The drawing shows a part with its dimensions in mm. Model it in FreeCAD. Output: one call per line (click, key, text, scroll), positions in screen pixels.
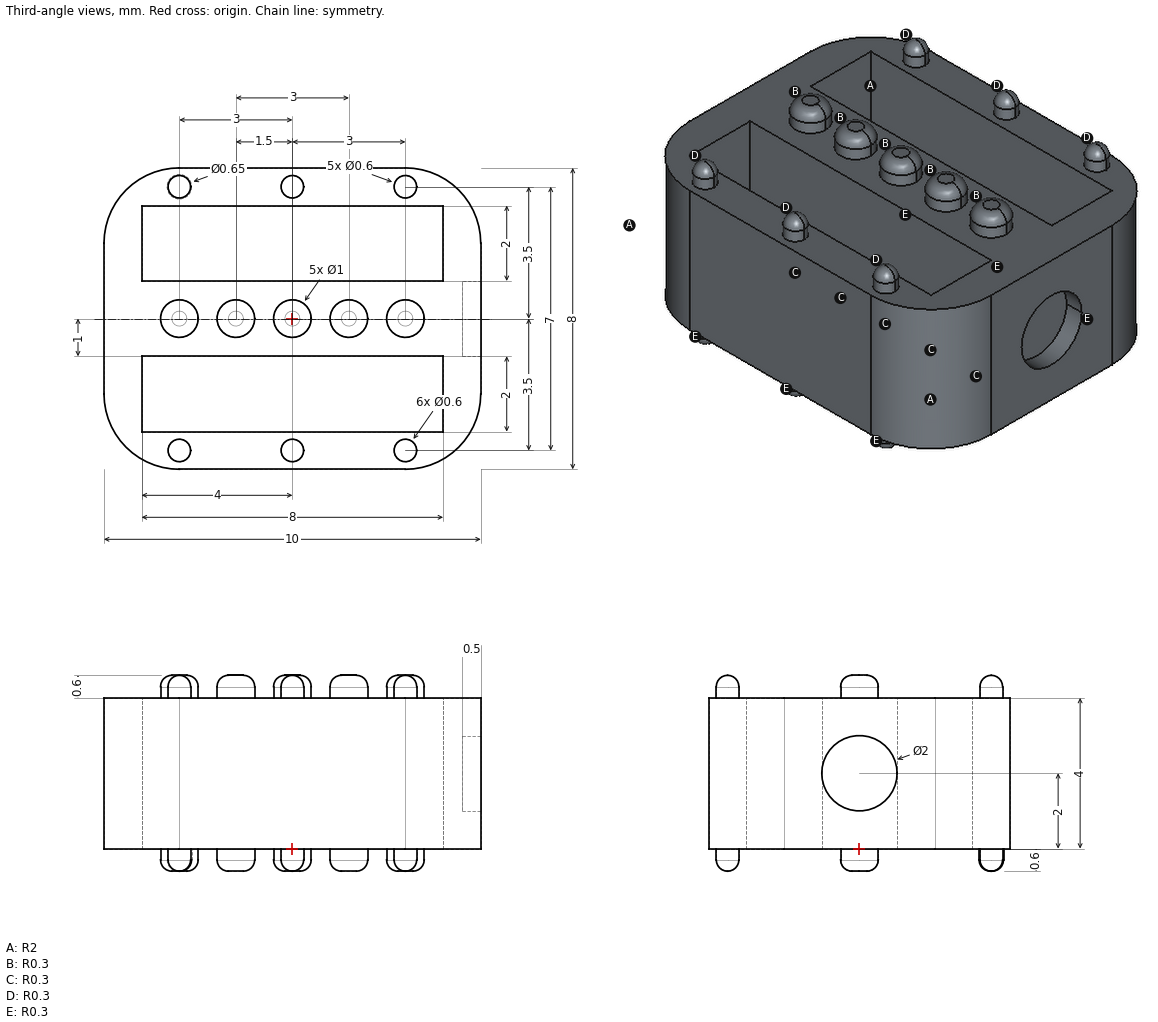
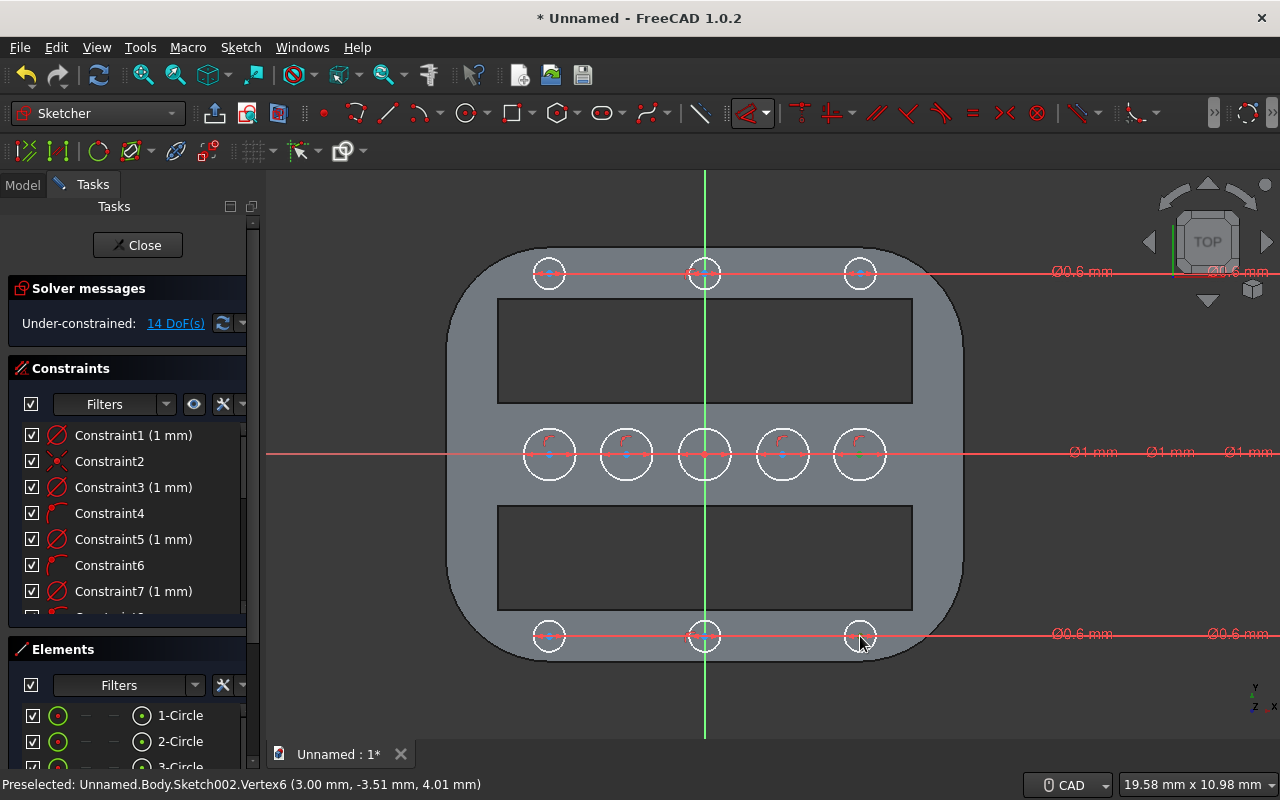
click(854, 114)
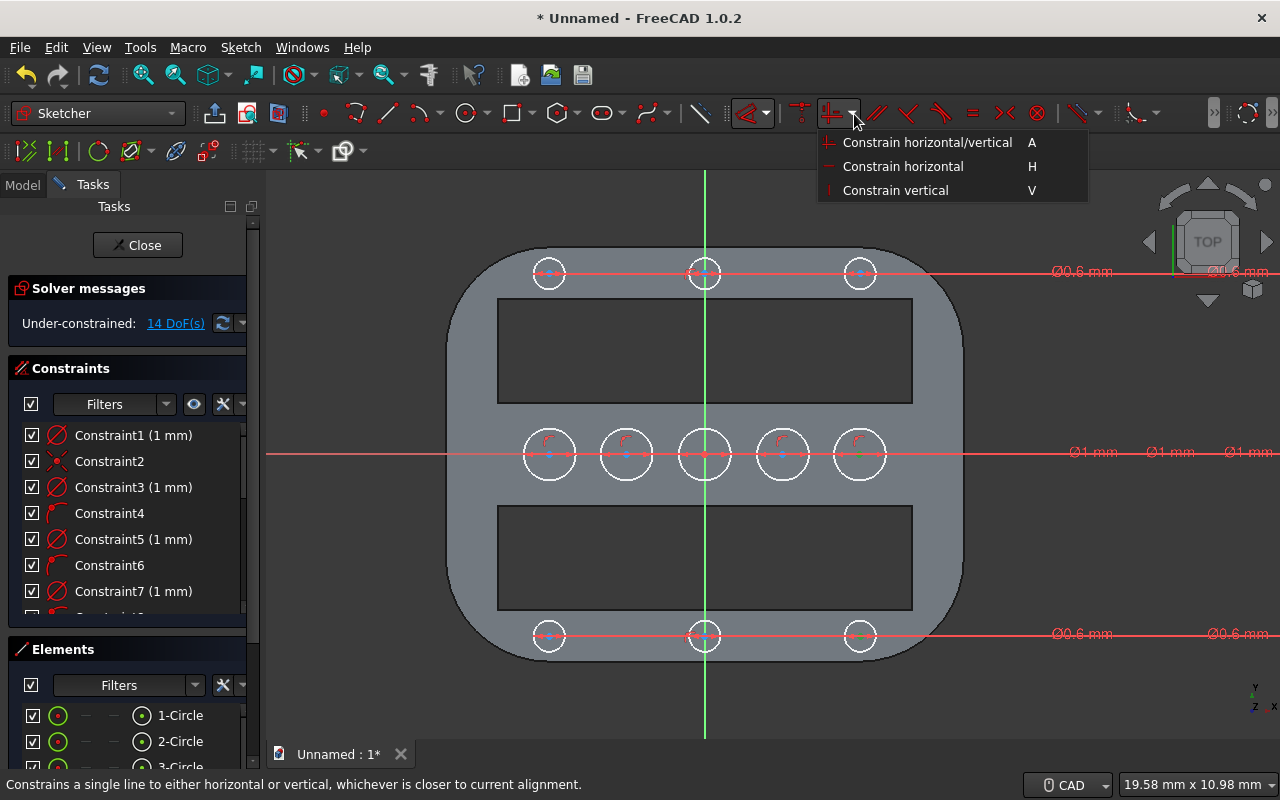
click(953, 190)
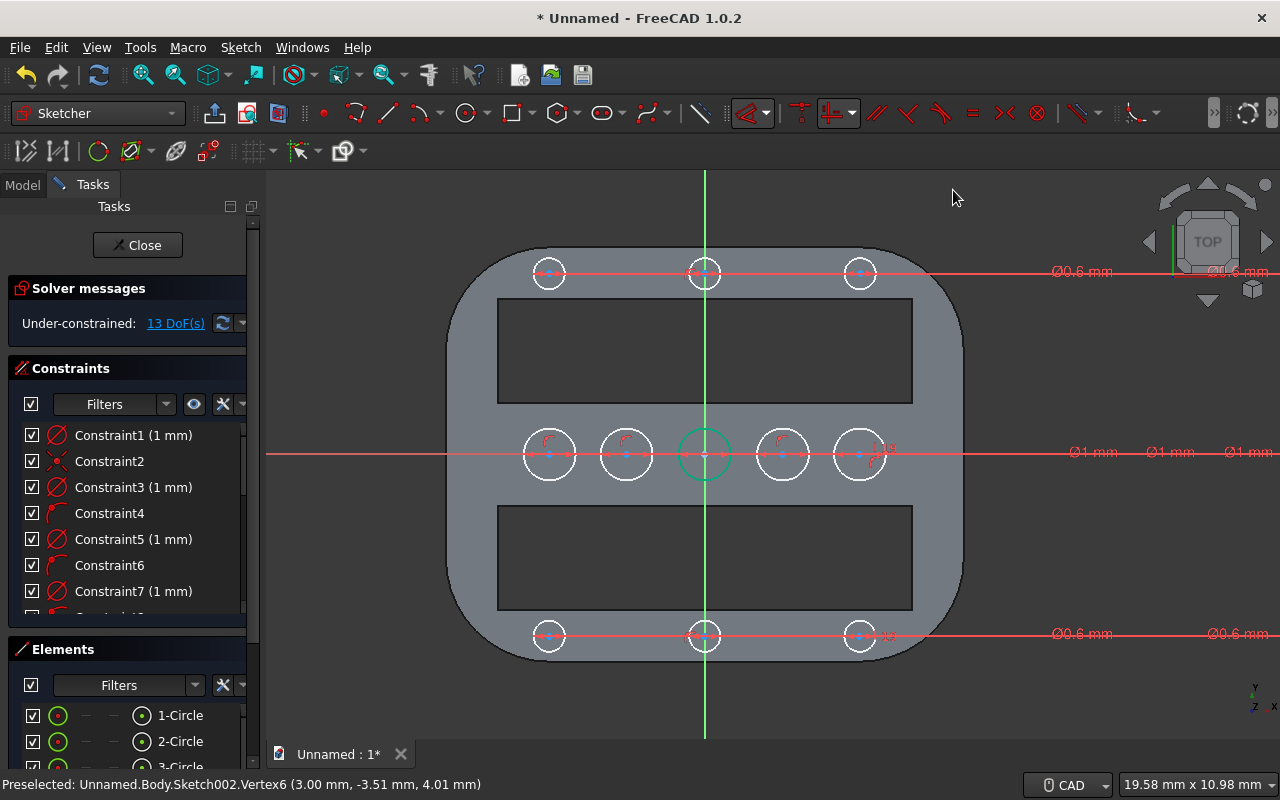
click(860, 636)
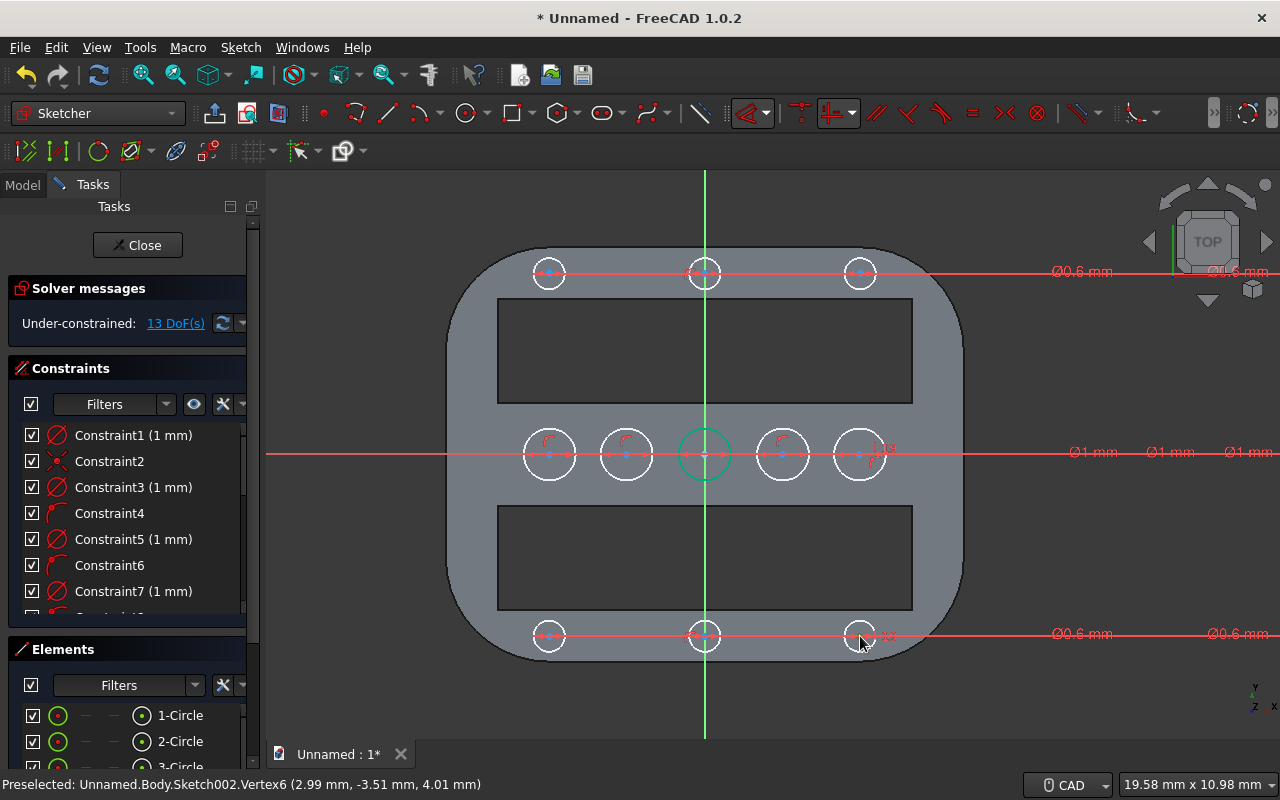
click(705, 636)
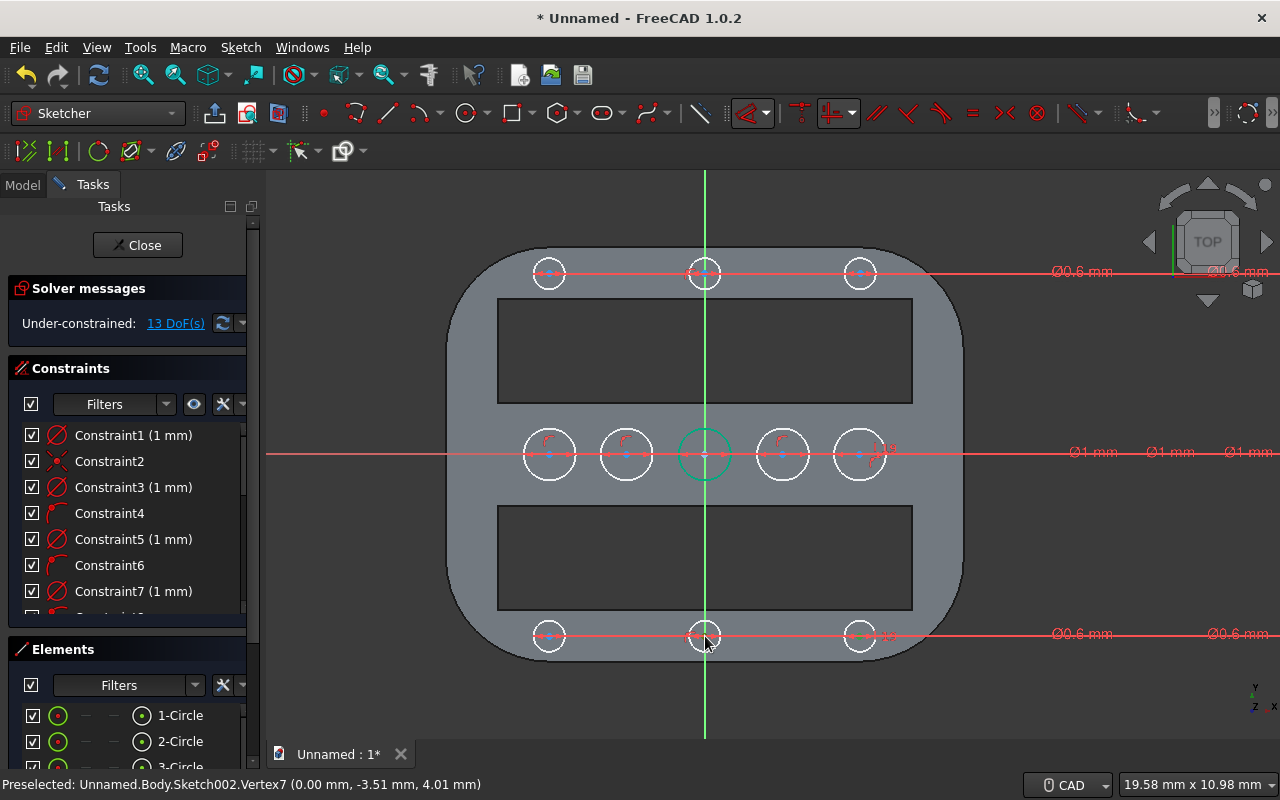
click(854, 114)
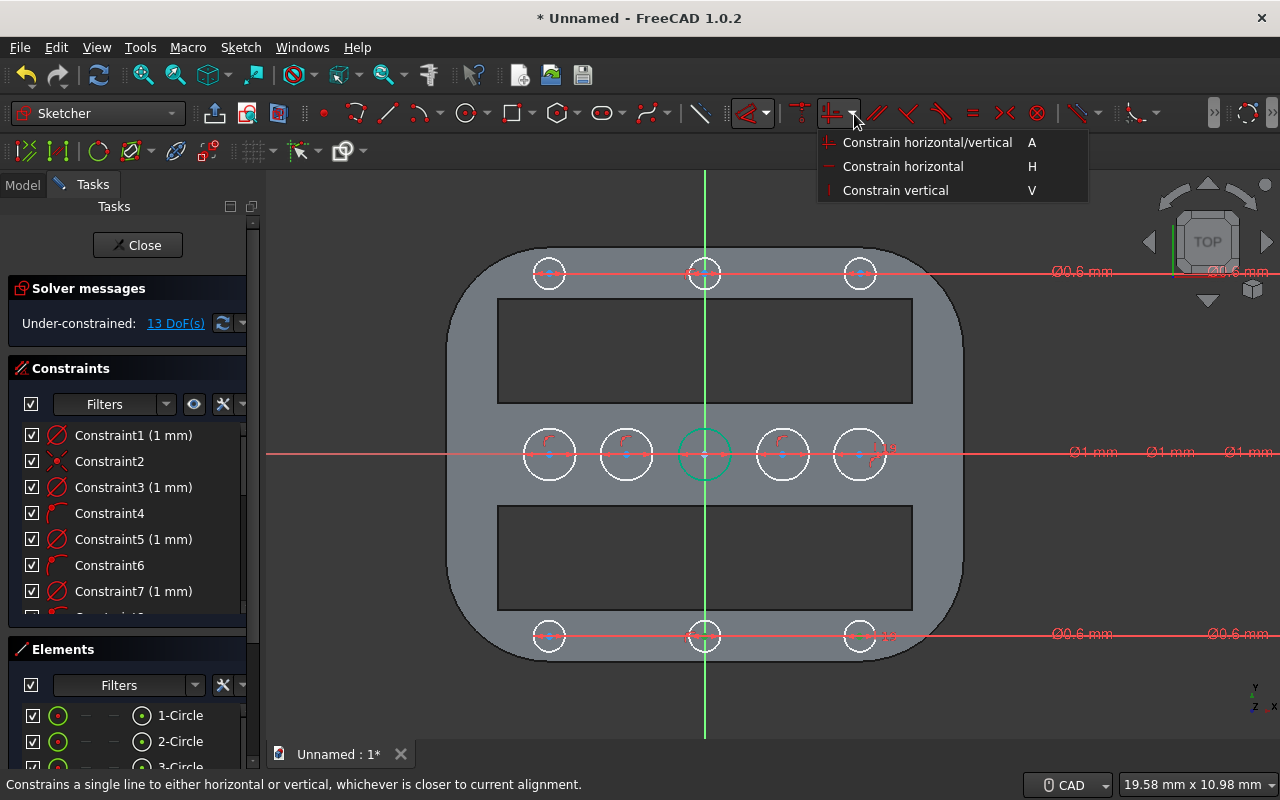
click(953, 166)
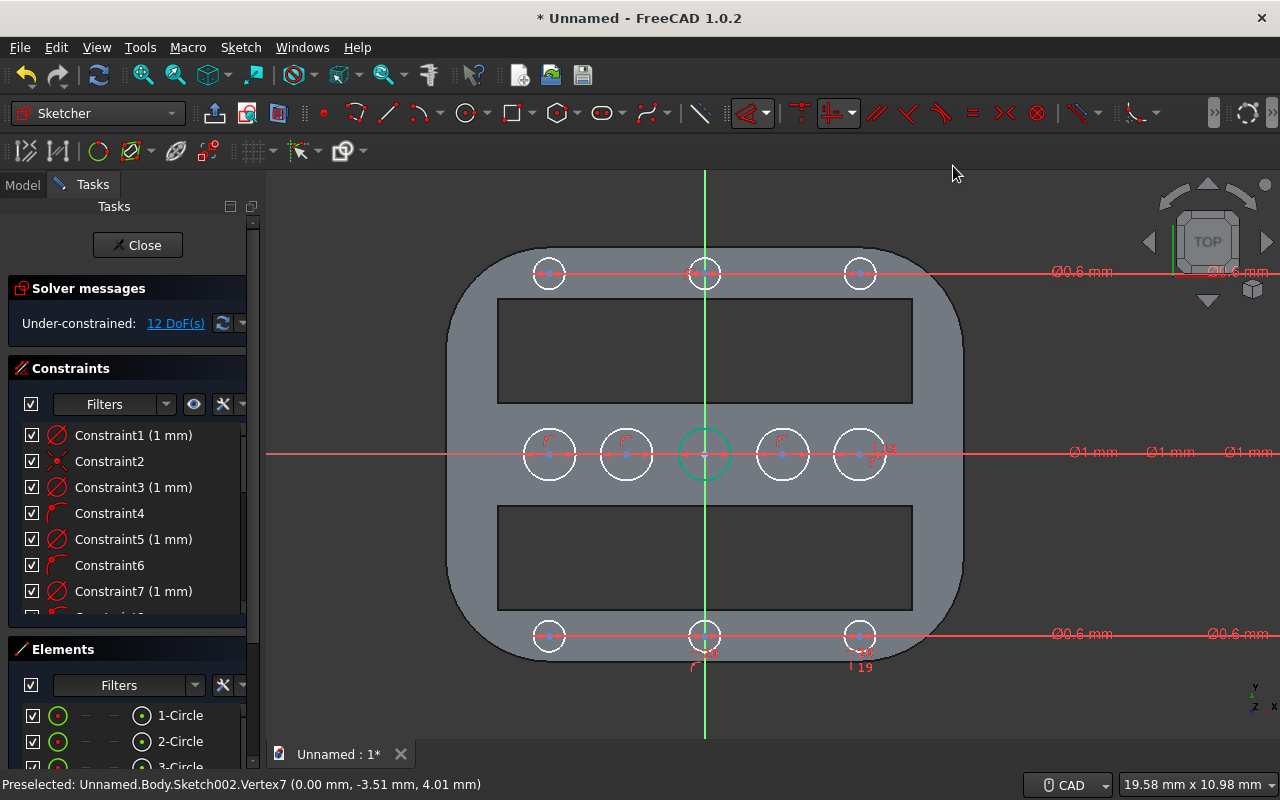
click(550, 454)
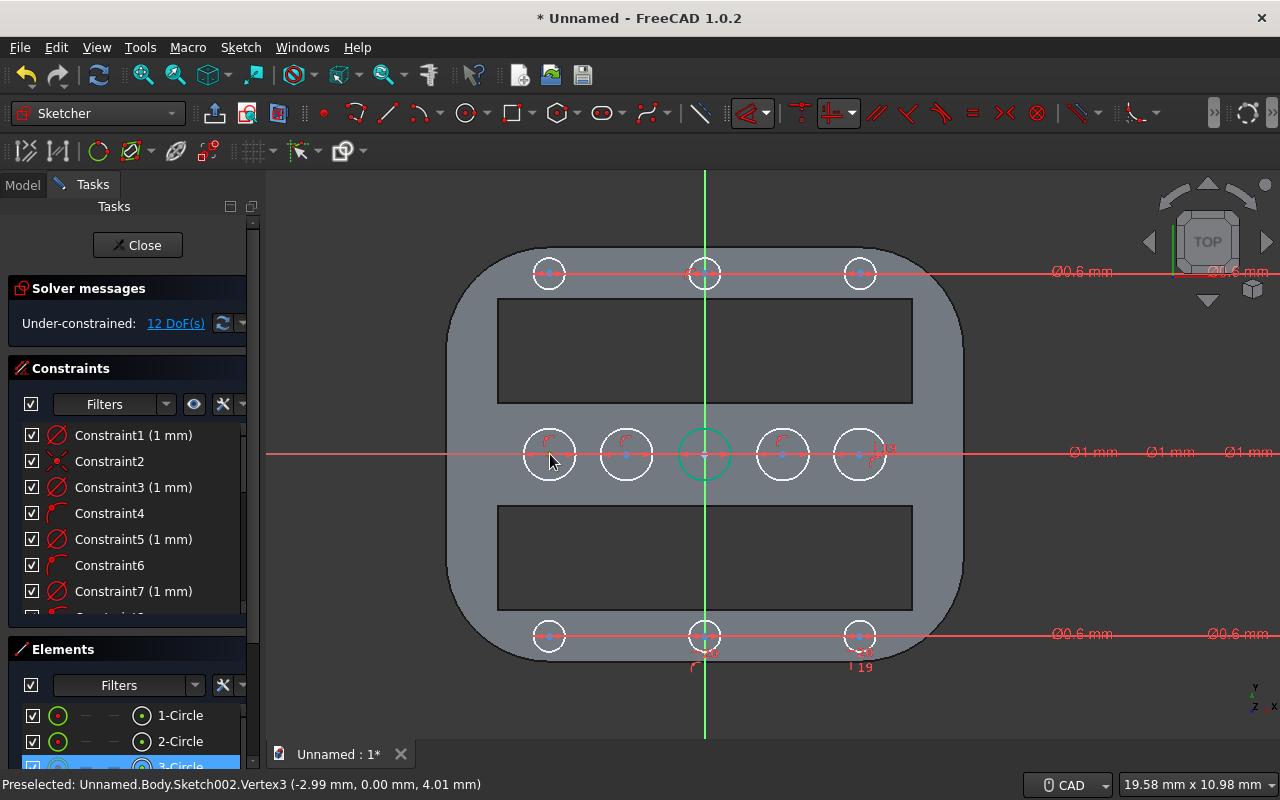
click(549, 636)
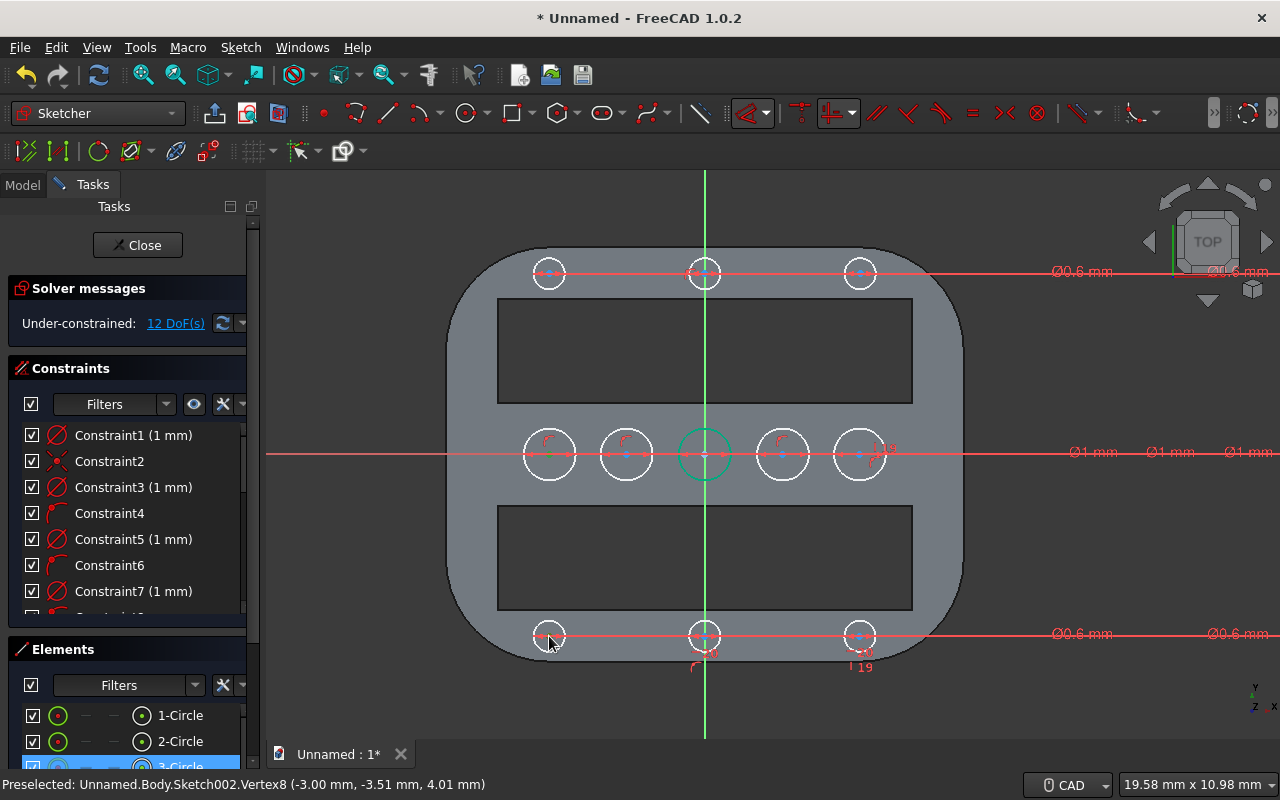
click(854, 114)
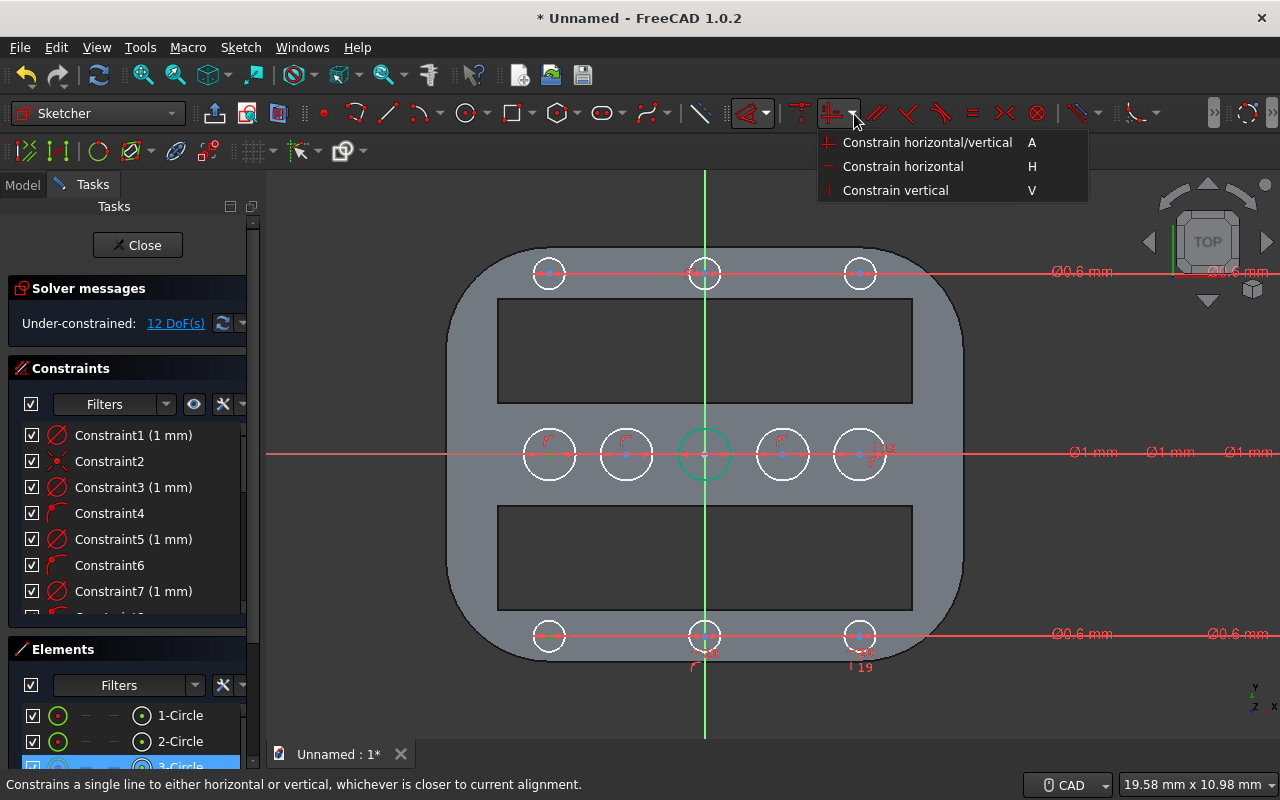
click(953, 190)